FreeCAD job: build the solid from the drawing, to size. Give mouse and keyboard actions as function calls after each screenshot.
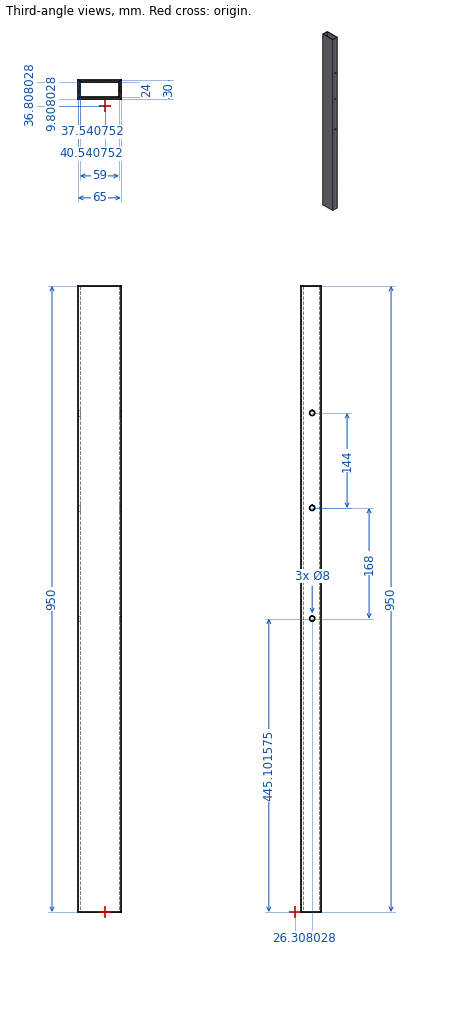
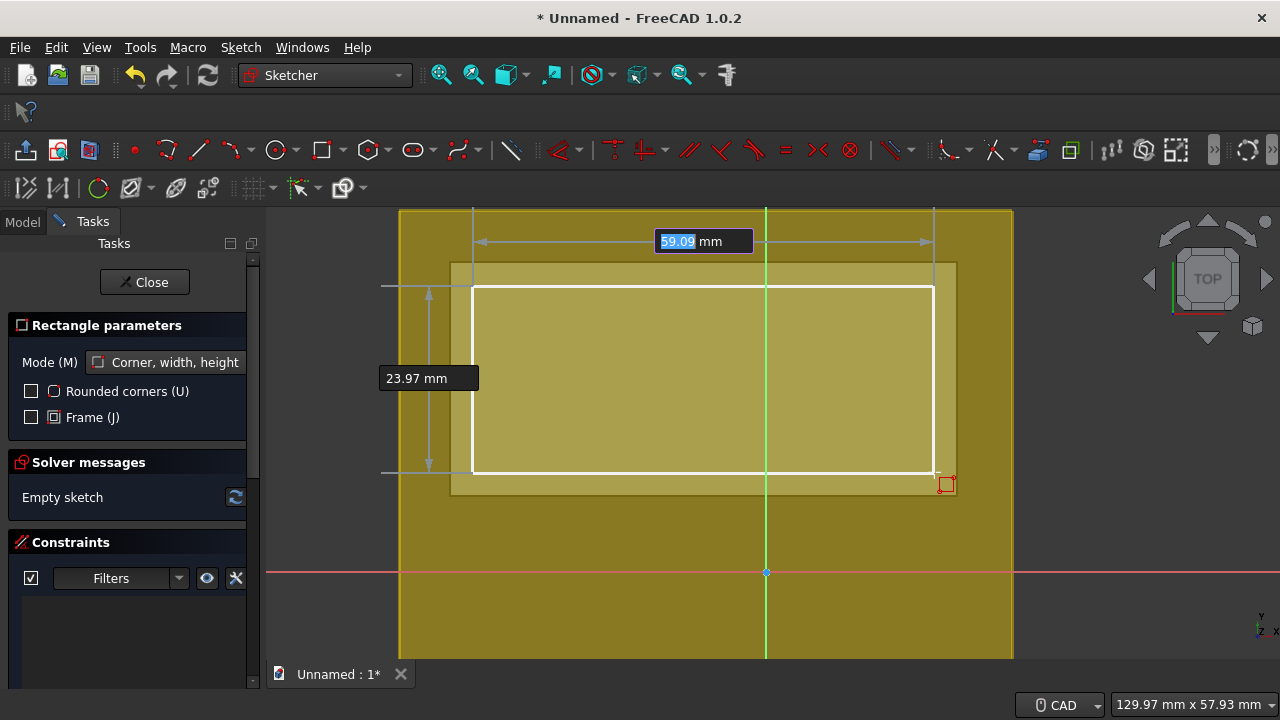
text(59)
key(Tab)
text(24)
key(Return)
key(Escape)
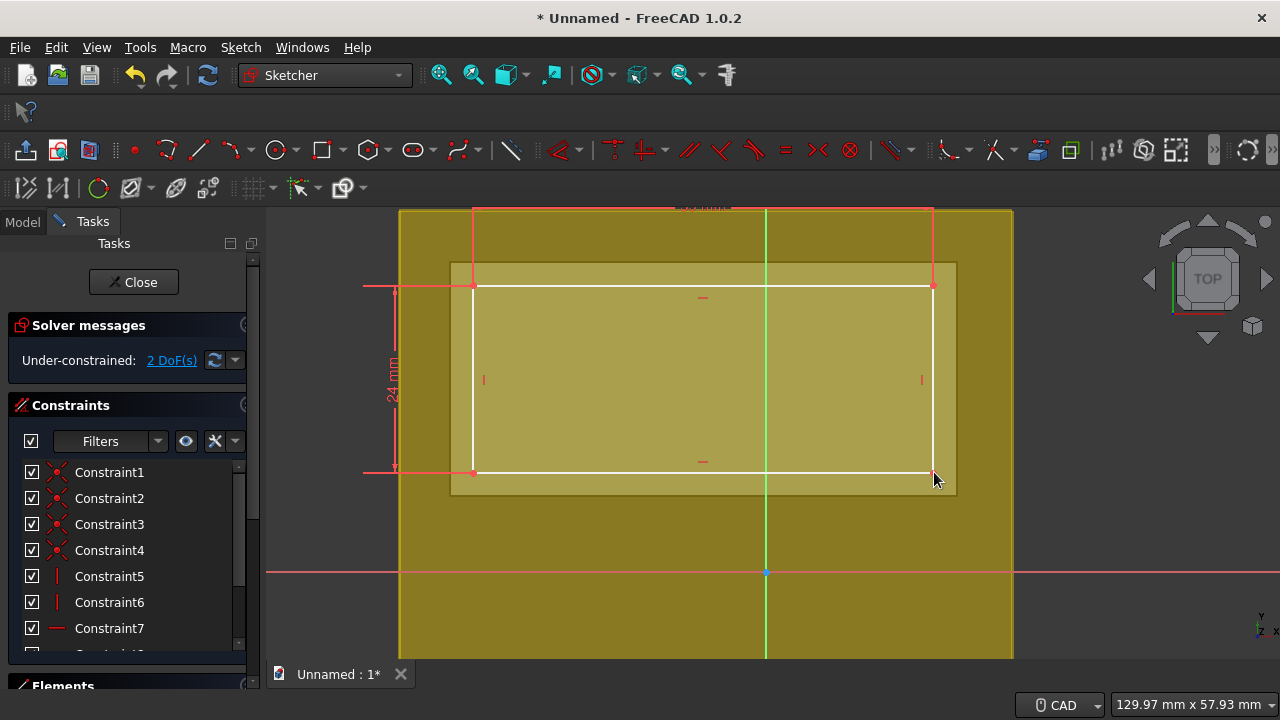
click(558, 150)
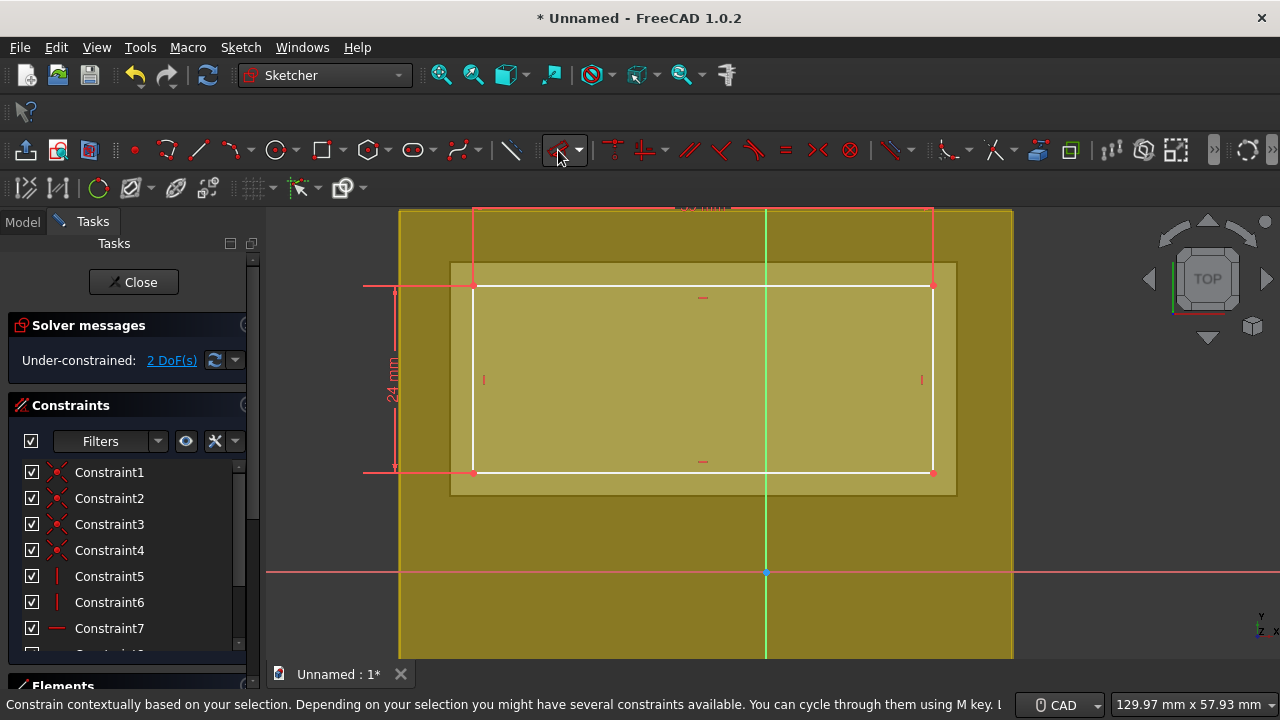
click(473, 286)
click(620, 606)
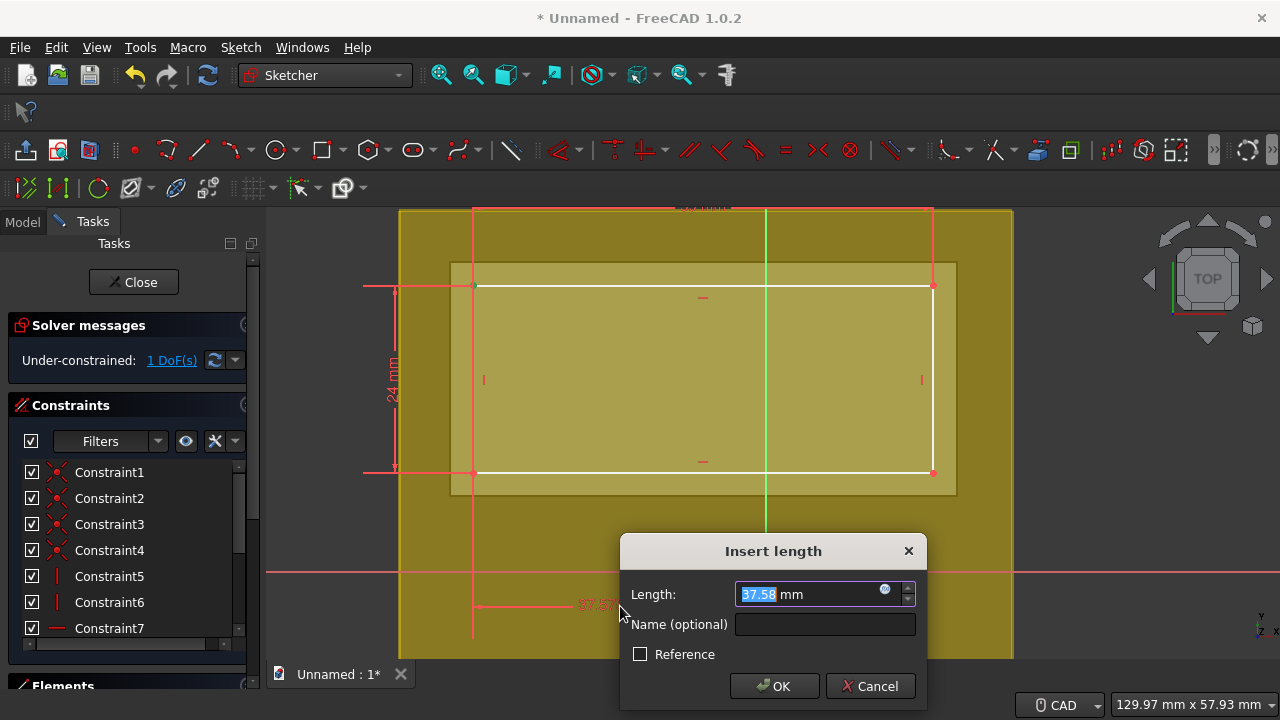
text(37.540752)
key(Return)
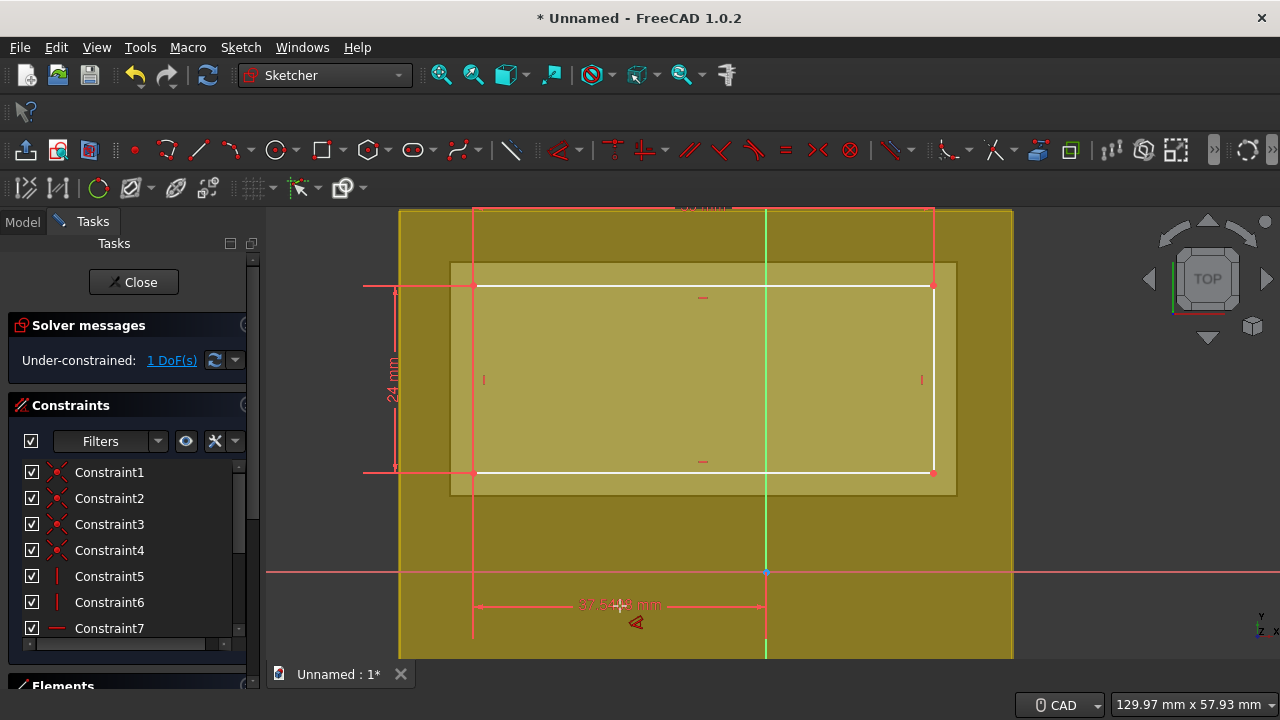
click(473, 286)
click(439, 429)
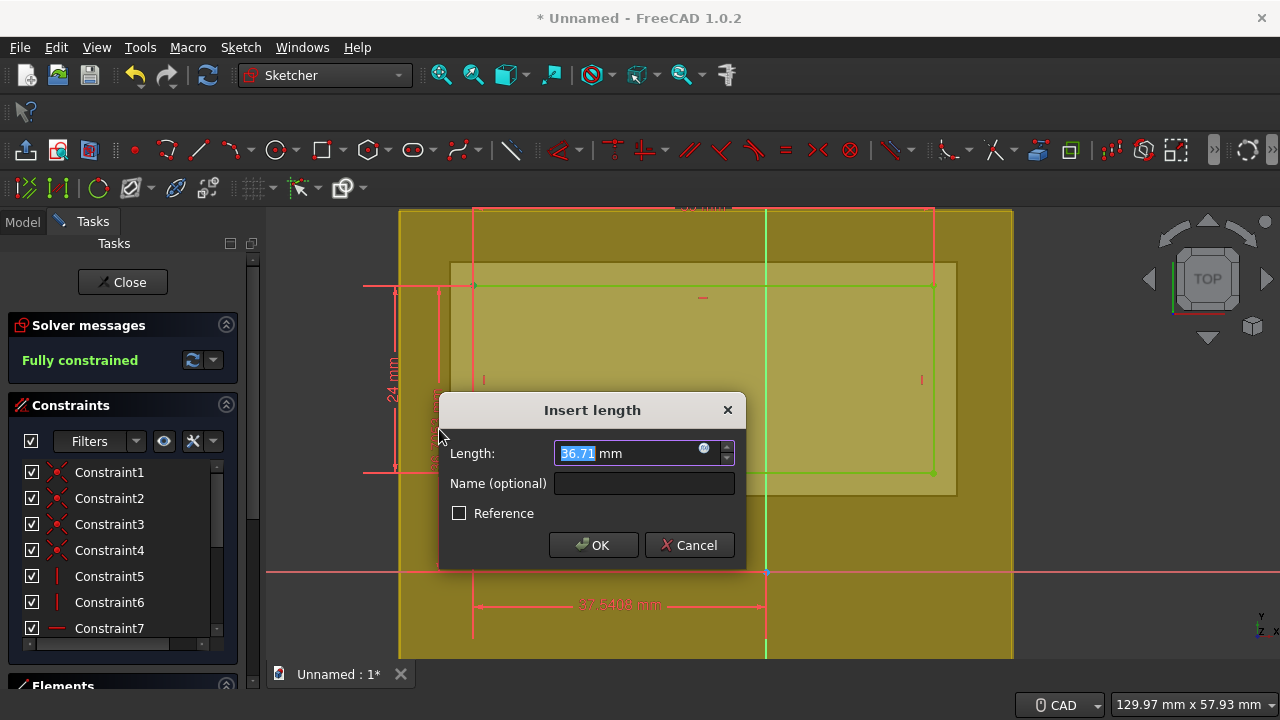
text(36.808028)
key(Return)
key(Escape)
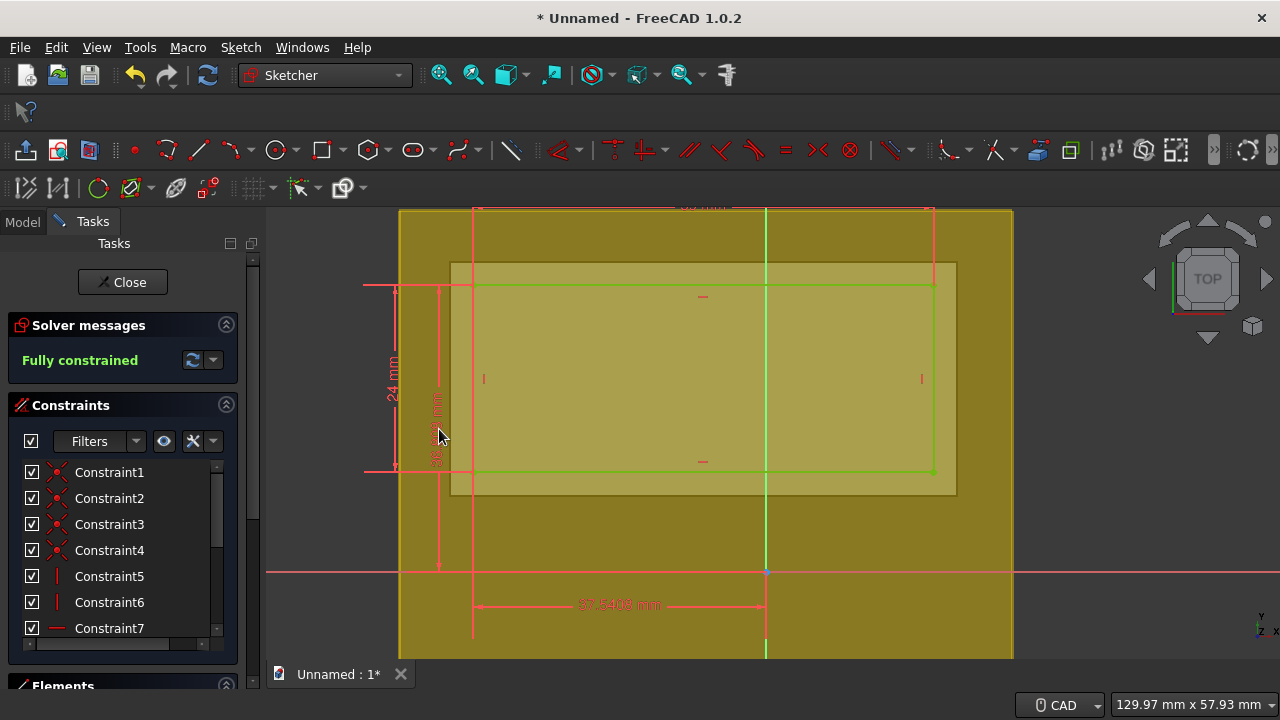
click(123, 282)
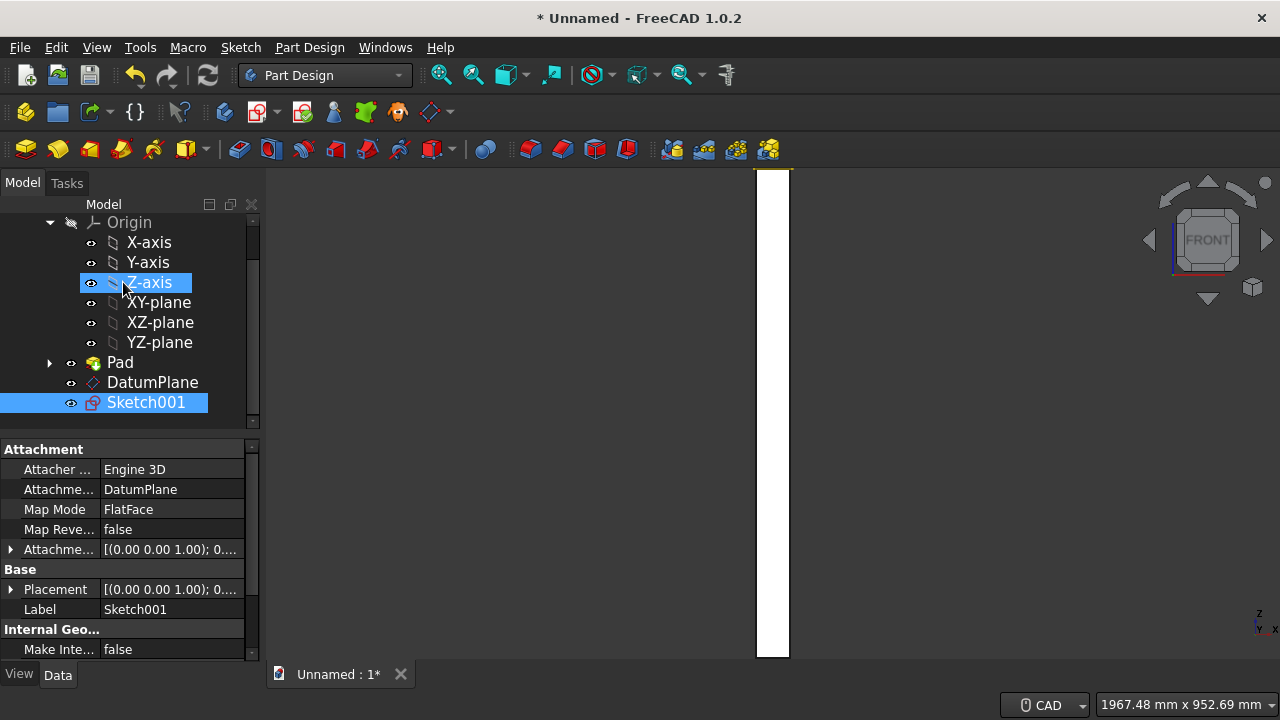
click(240, 150)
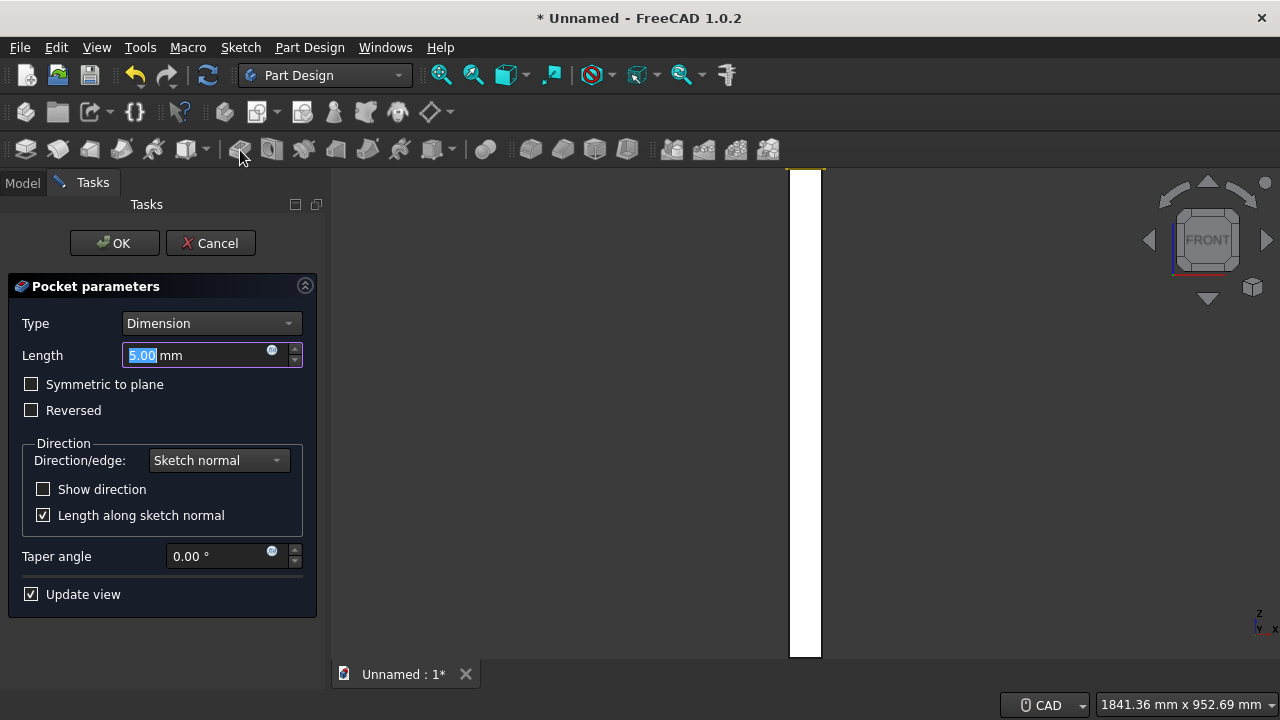
text(950)
key(Tab)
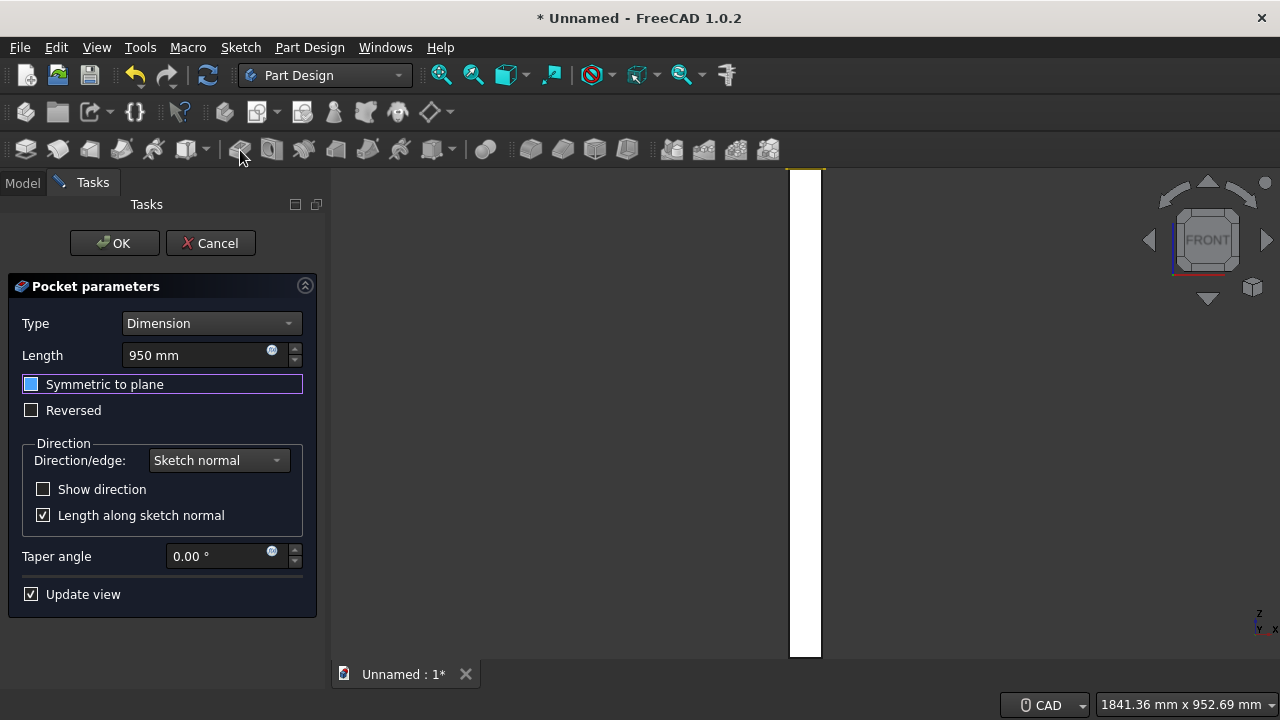
click(115, 243)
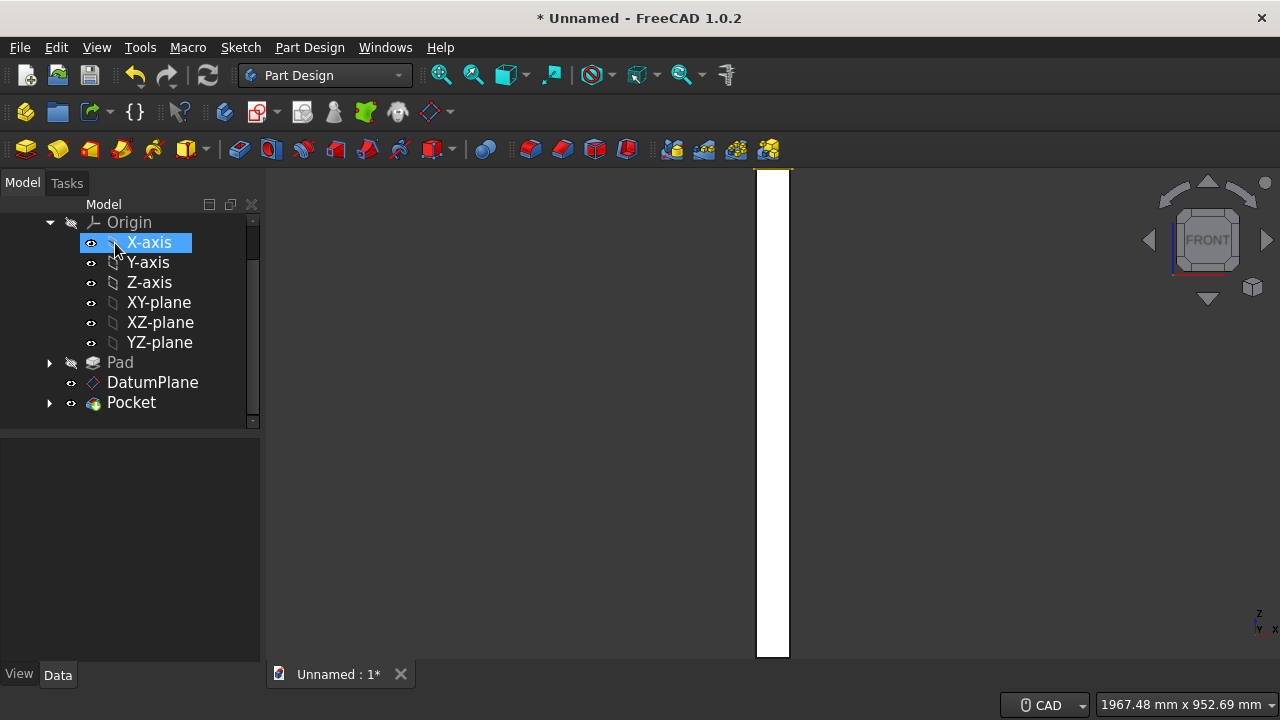
click(116, 383)
key(space)